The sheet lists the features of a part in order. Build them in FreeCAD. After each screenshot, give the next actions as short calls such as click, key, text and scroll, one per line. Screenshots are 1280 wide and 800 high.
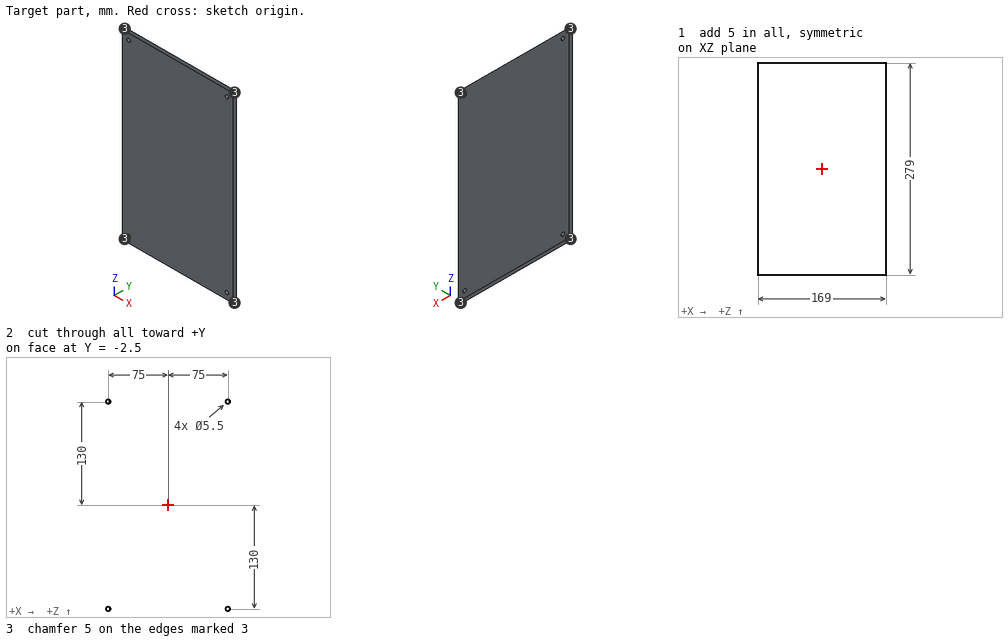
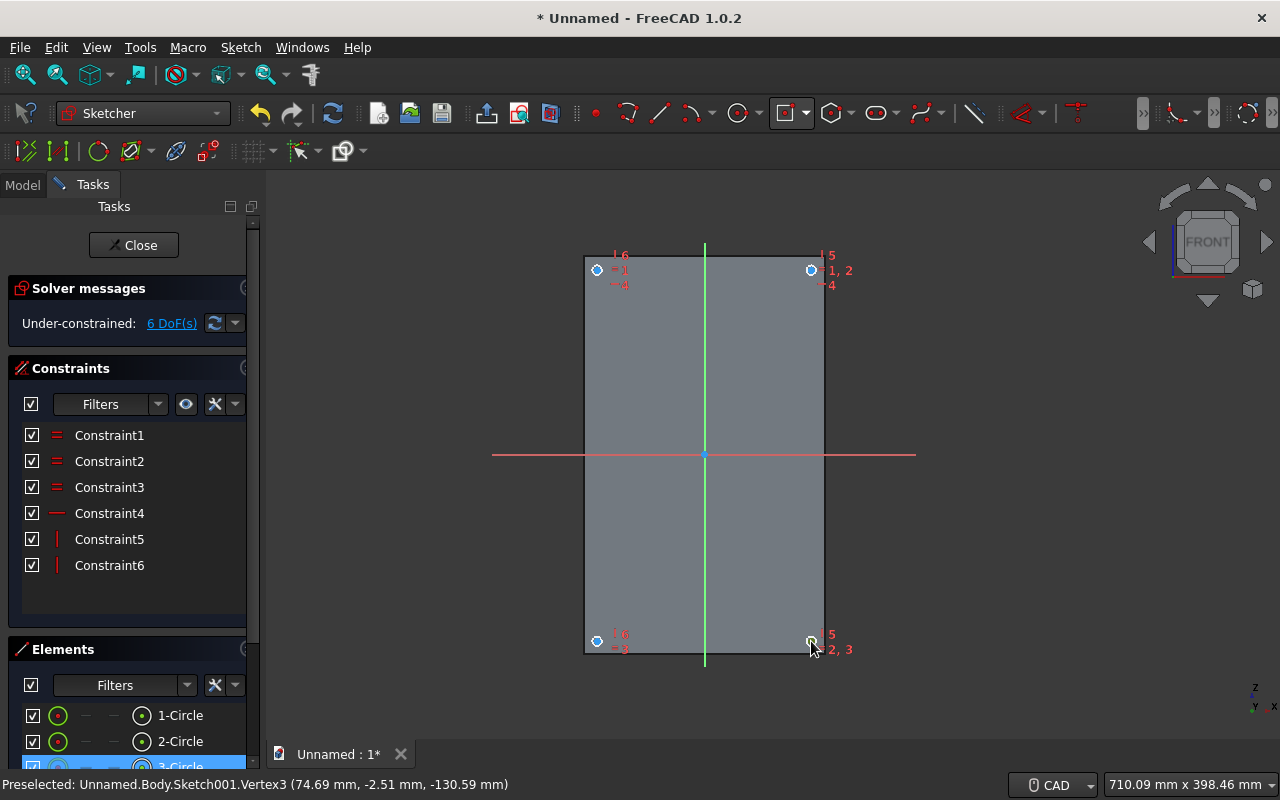
click(597, 641)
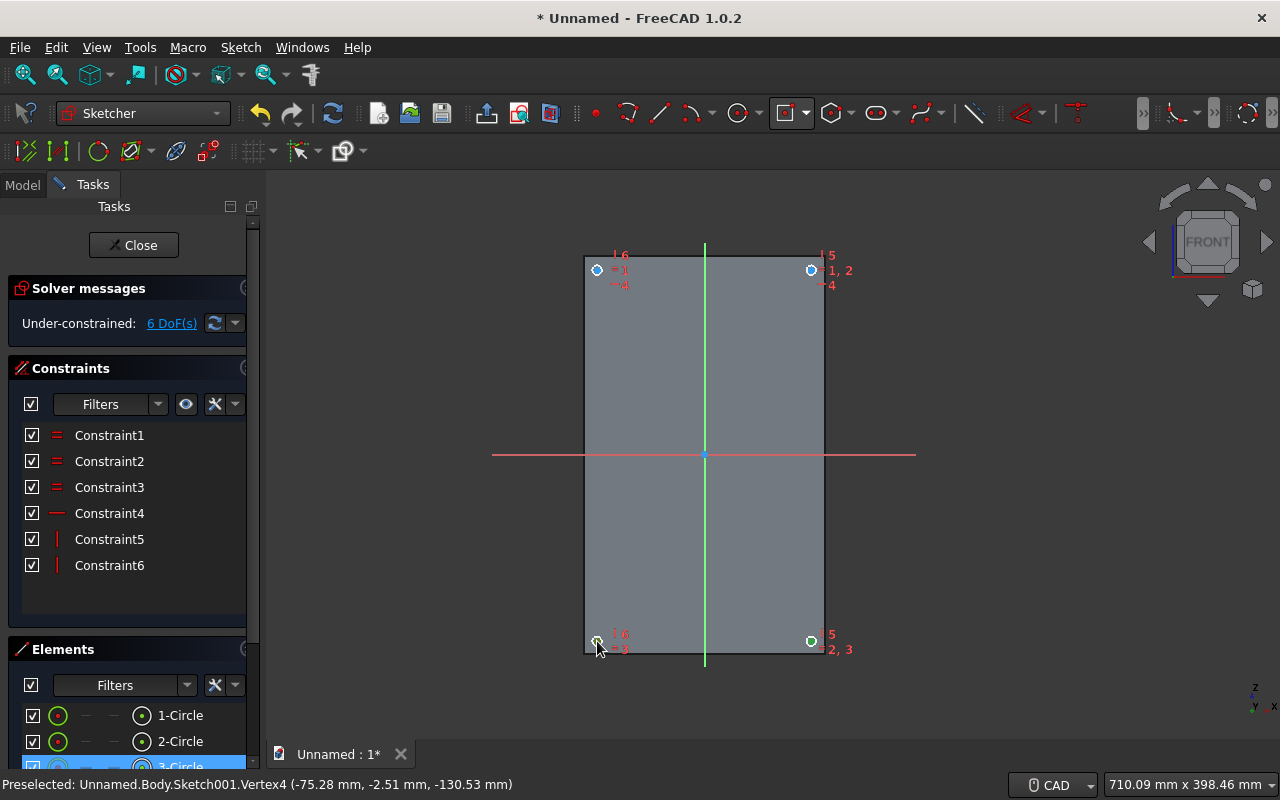
key(h)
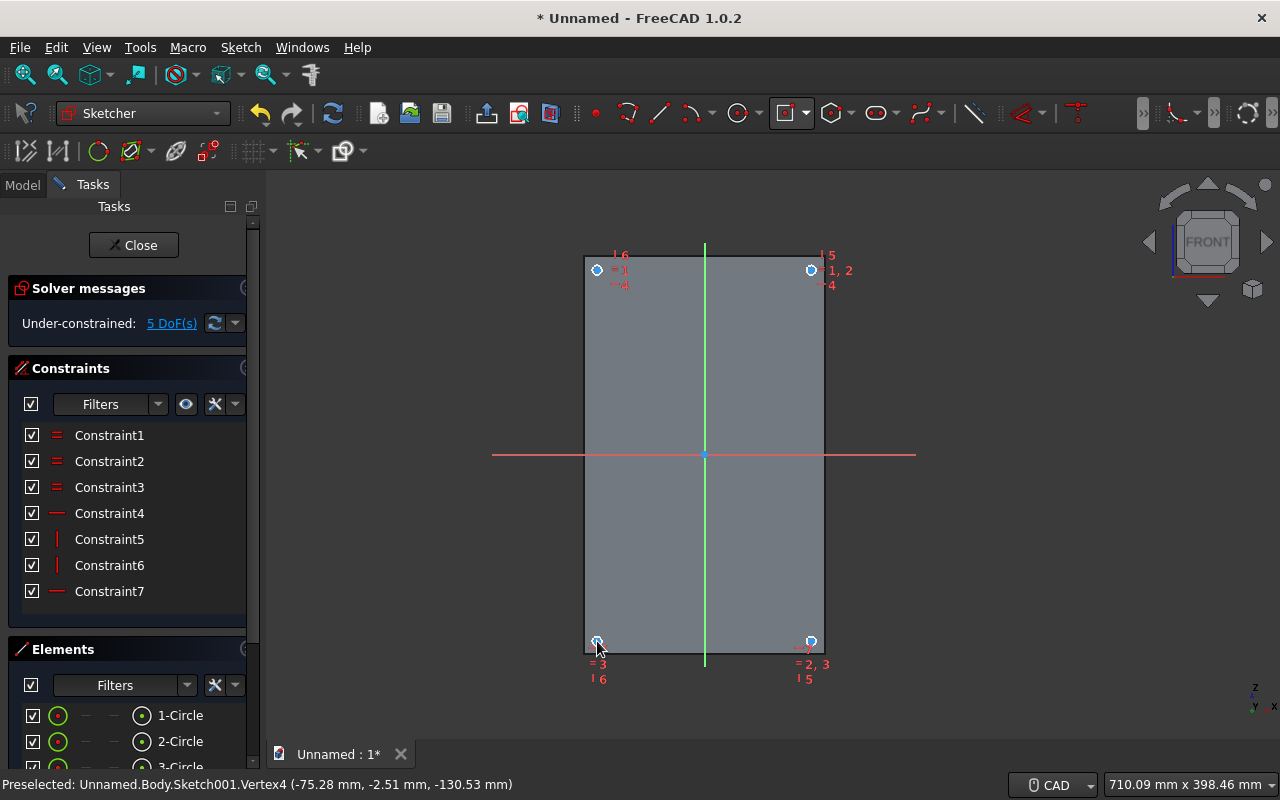
click(1022, 114)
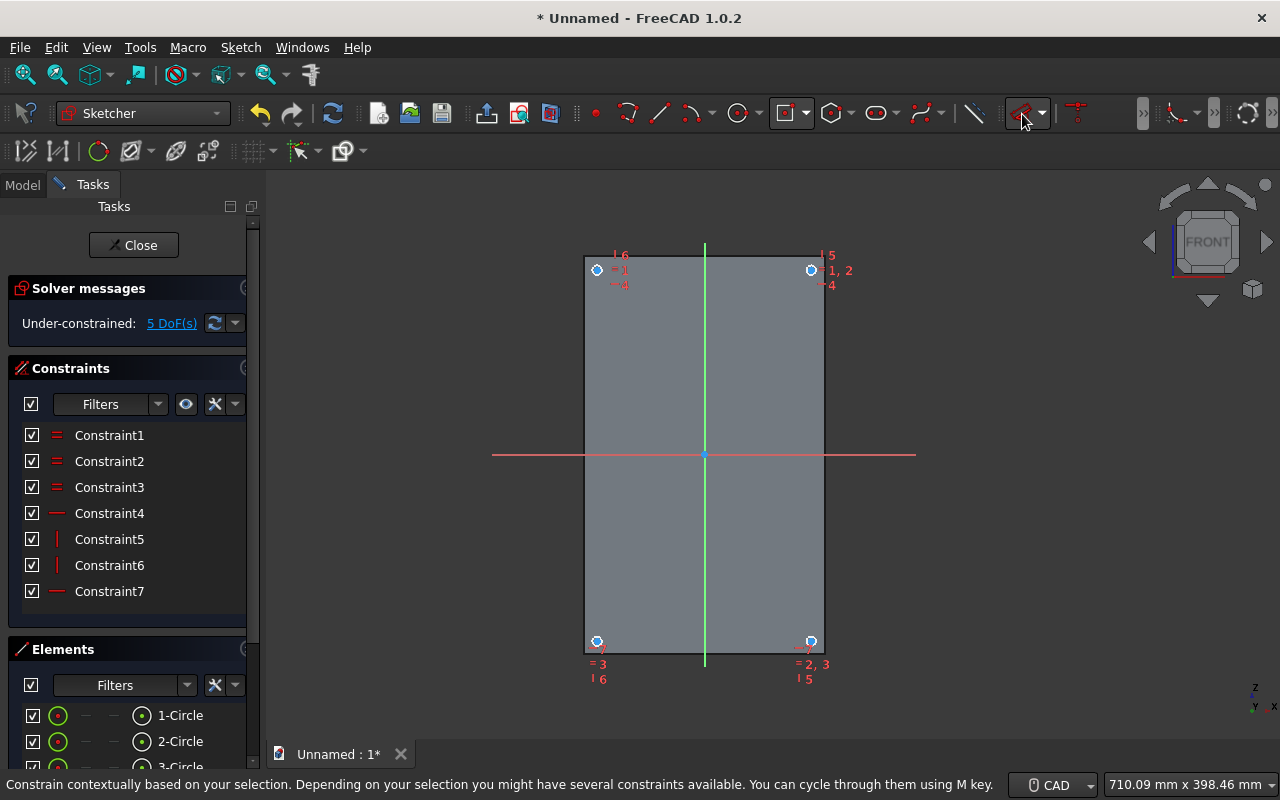
scroll(597, 265, up, 9)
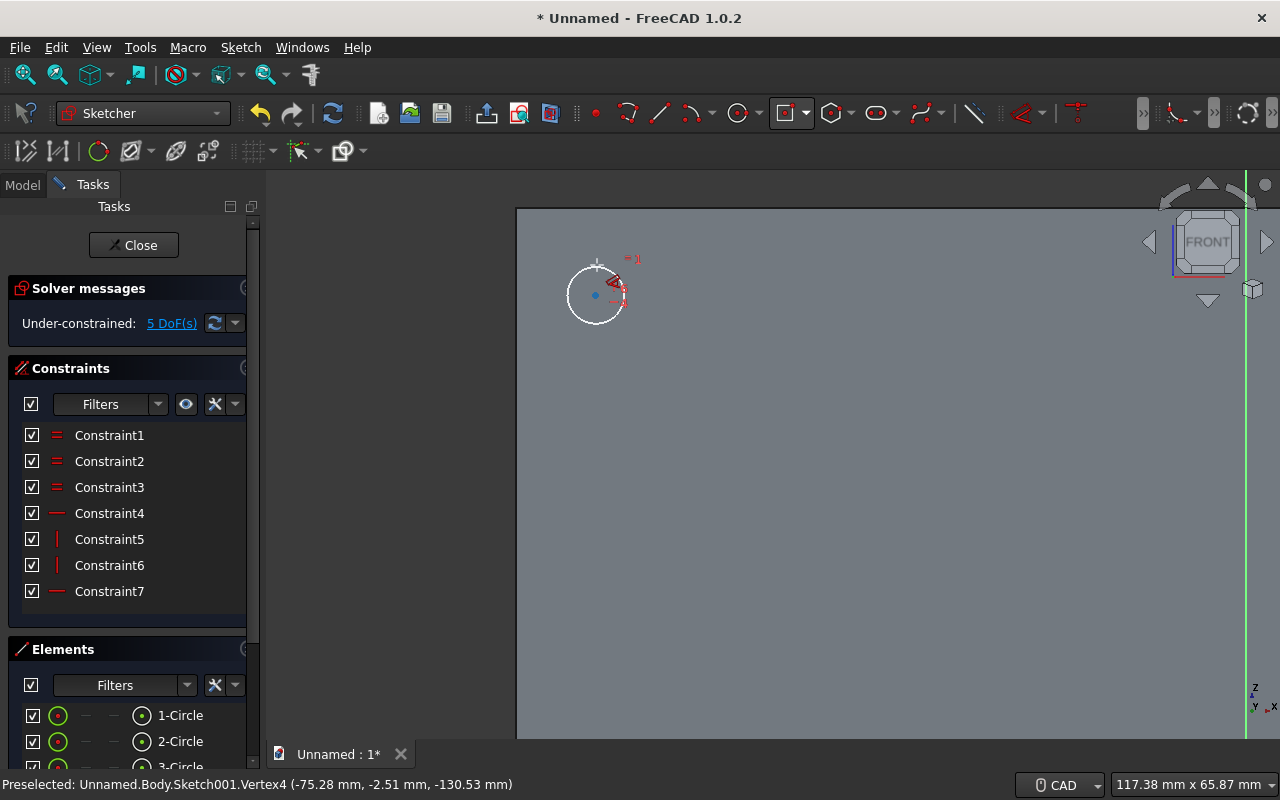
click(597, 267)
click(598, 235)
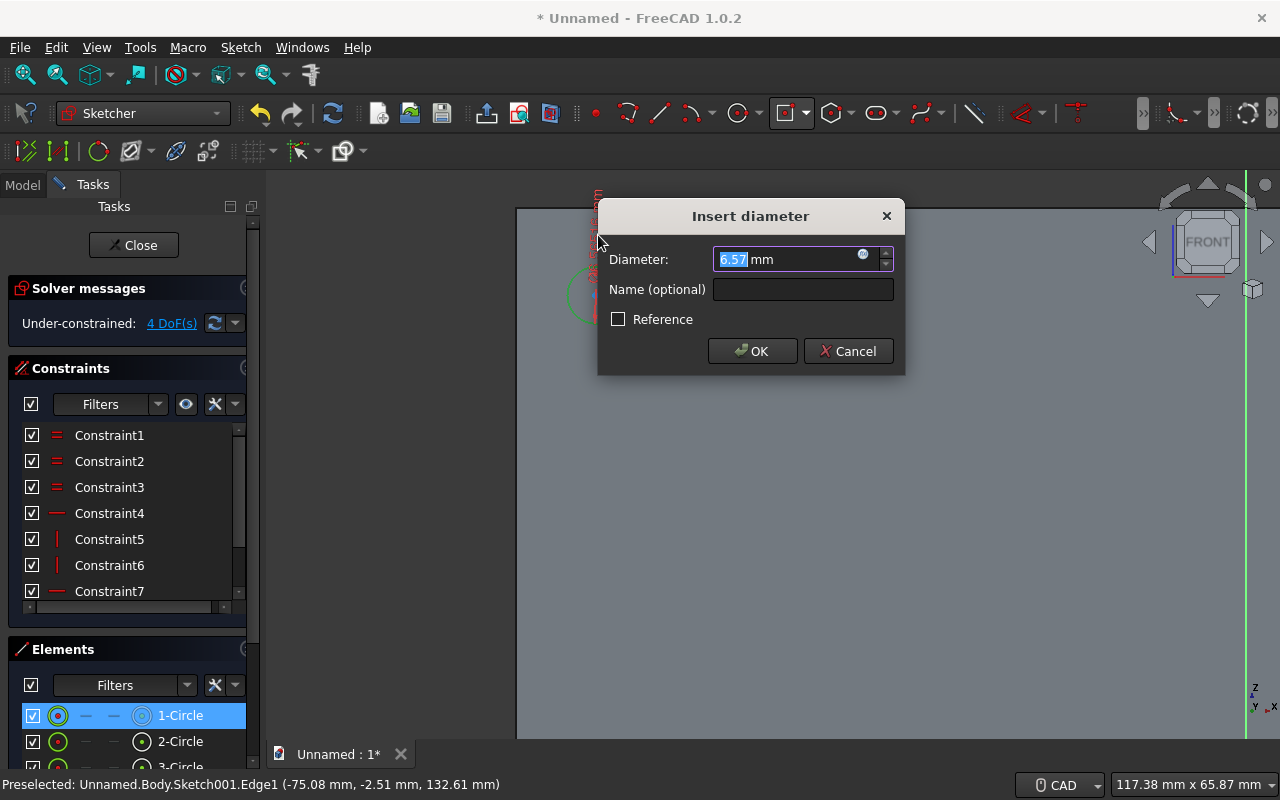
text(5.5)
key(Return)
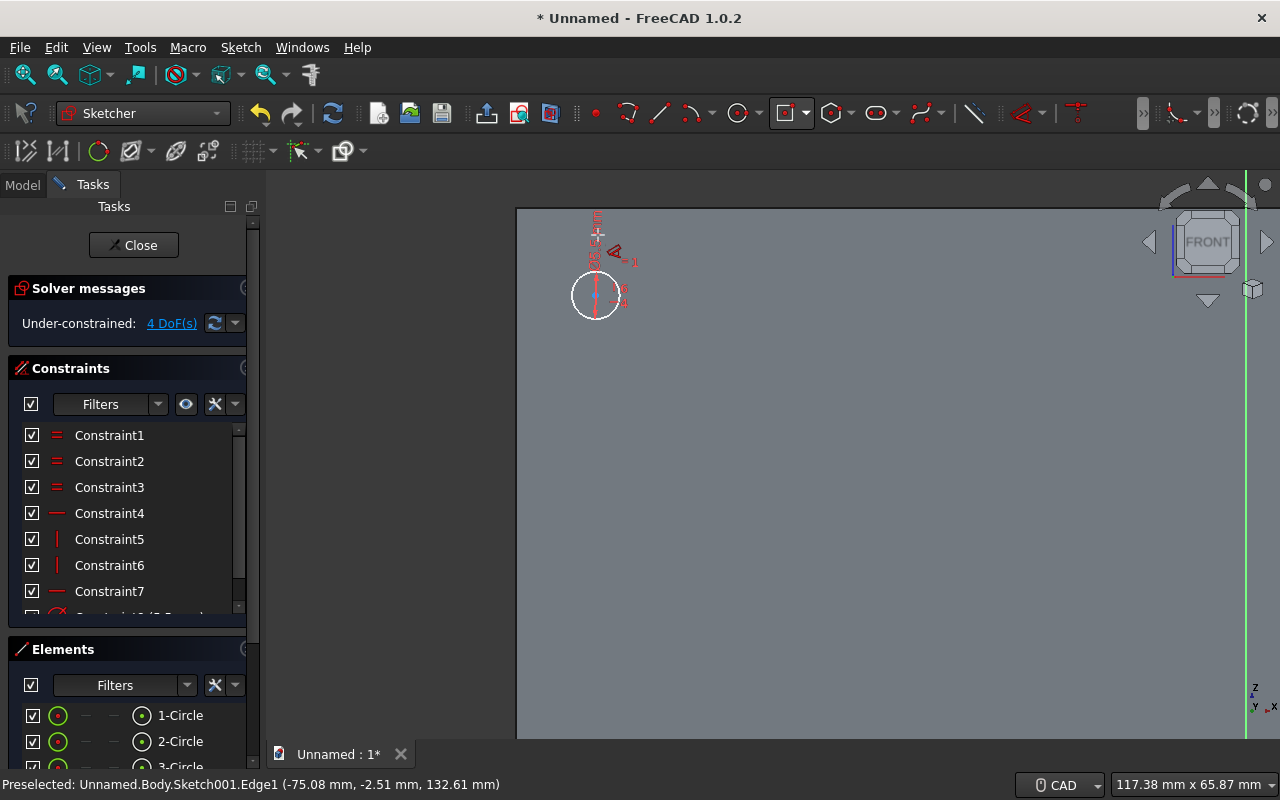
scroll(597, 265, down, 9)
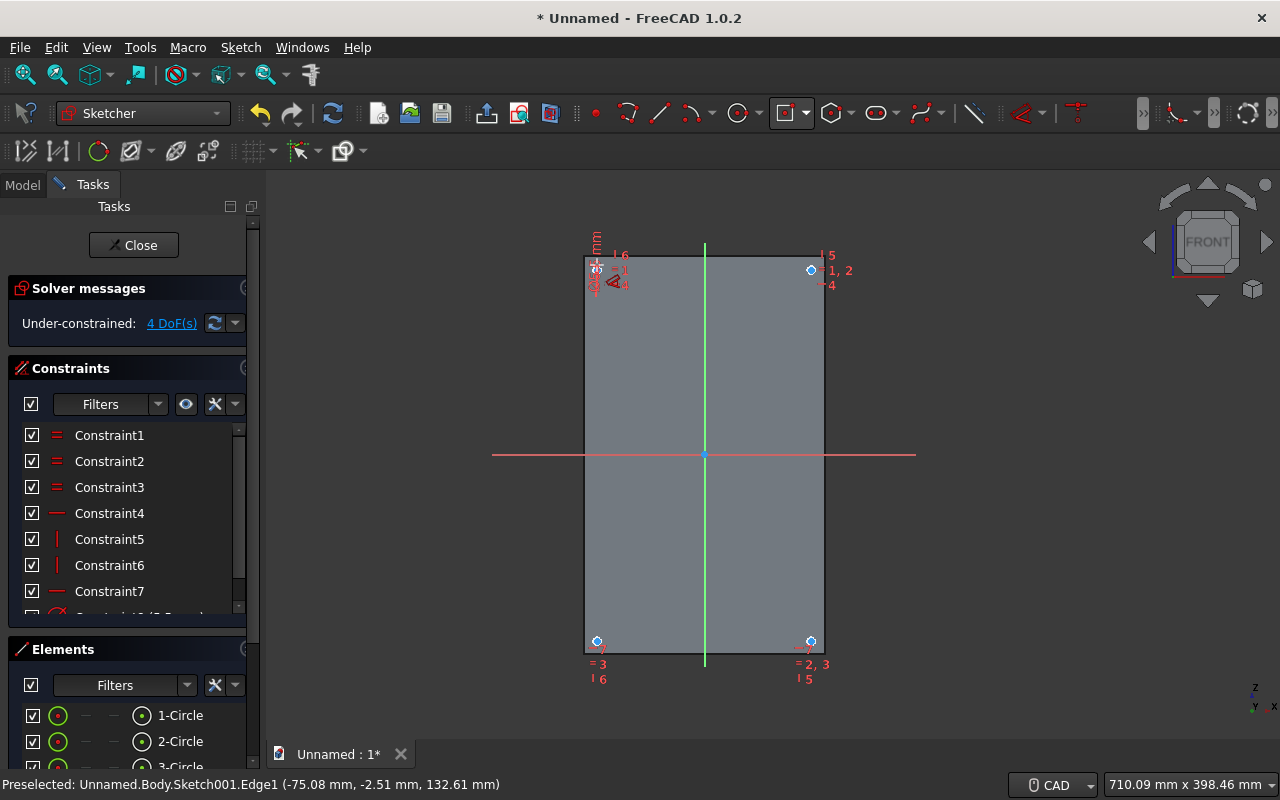
click(597, 270)
click(651, 236)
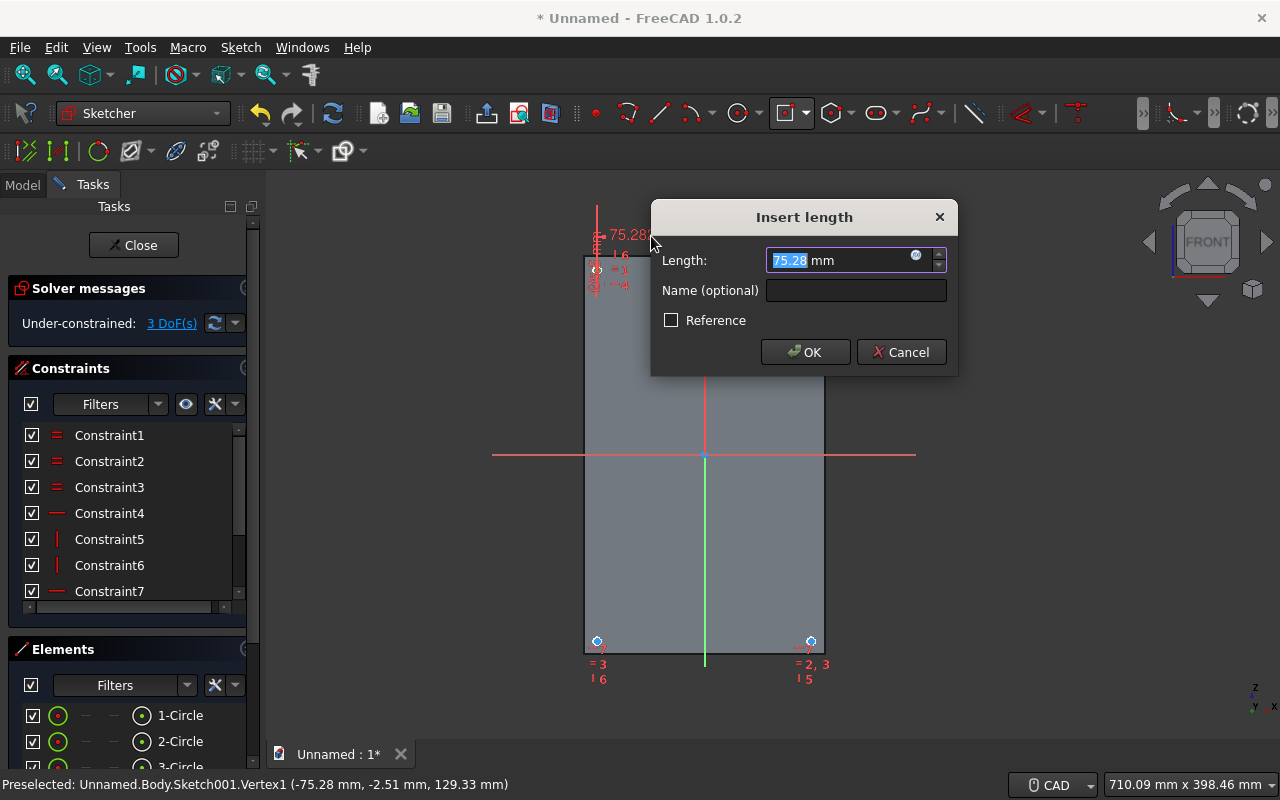
text(75)
key(Return)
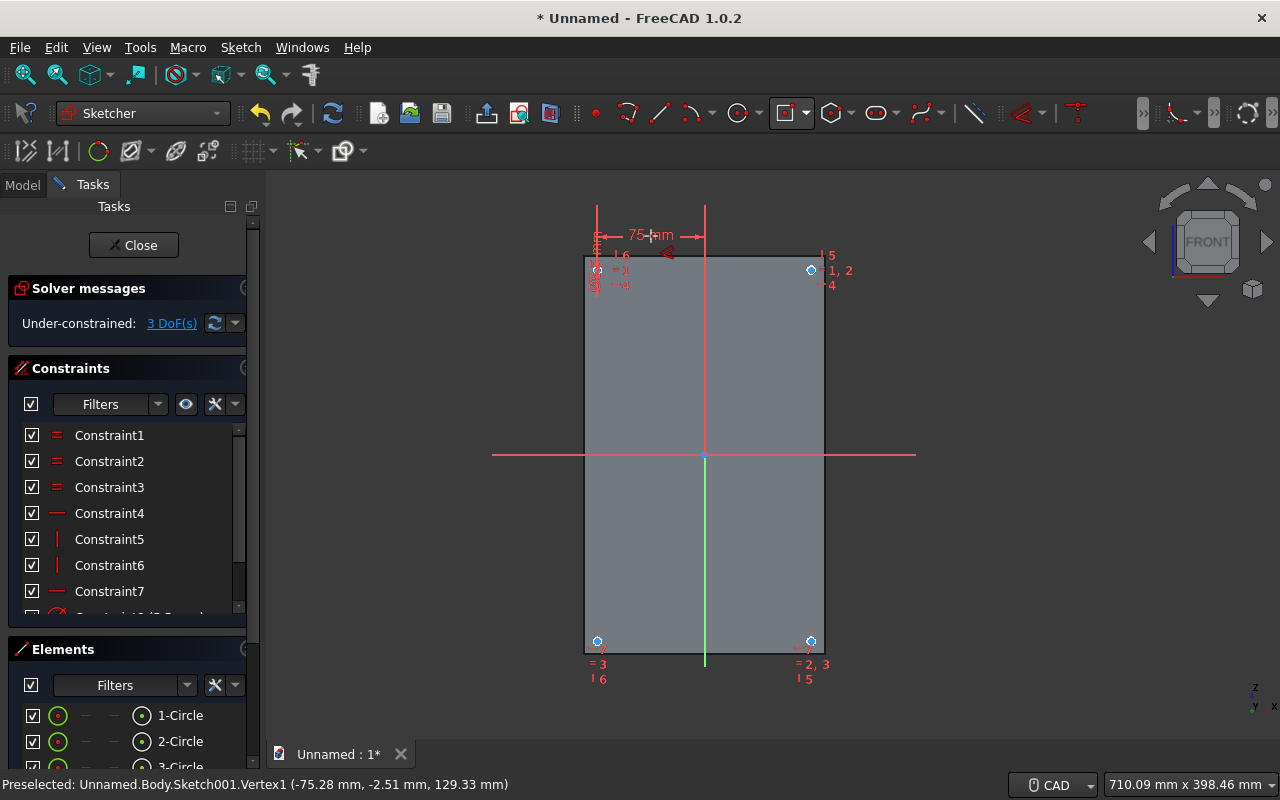
click(811, 270)
click(758, 236)